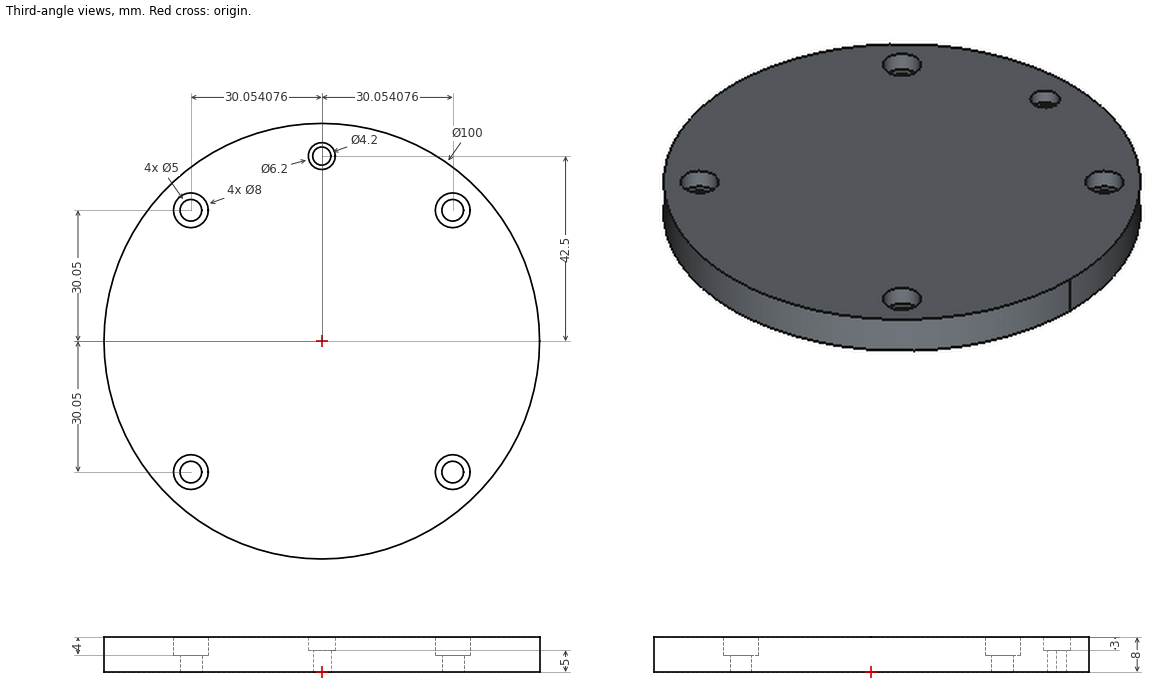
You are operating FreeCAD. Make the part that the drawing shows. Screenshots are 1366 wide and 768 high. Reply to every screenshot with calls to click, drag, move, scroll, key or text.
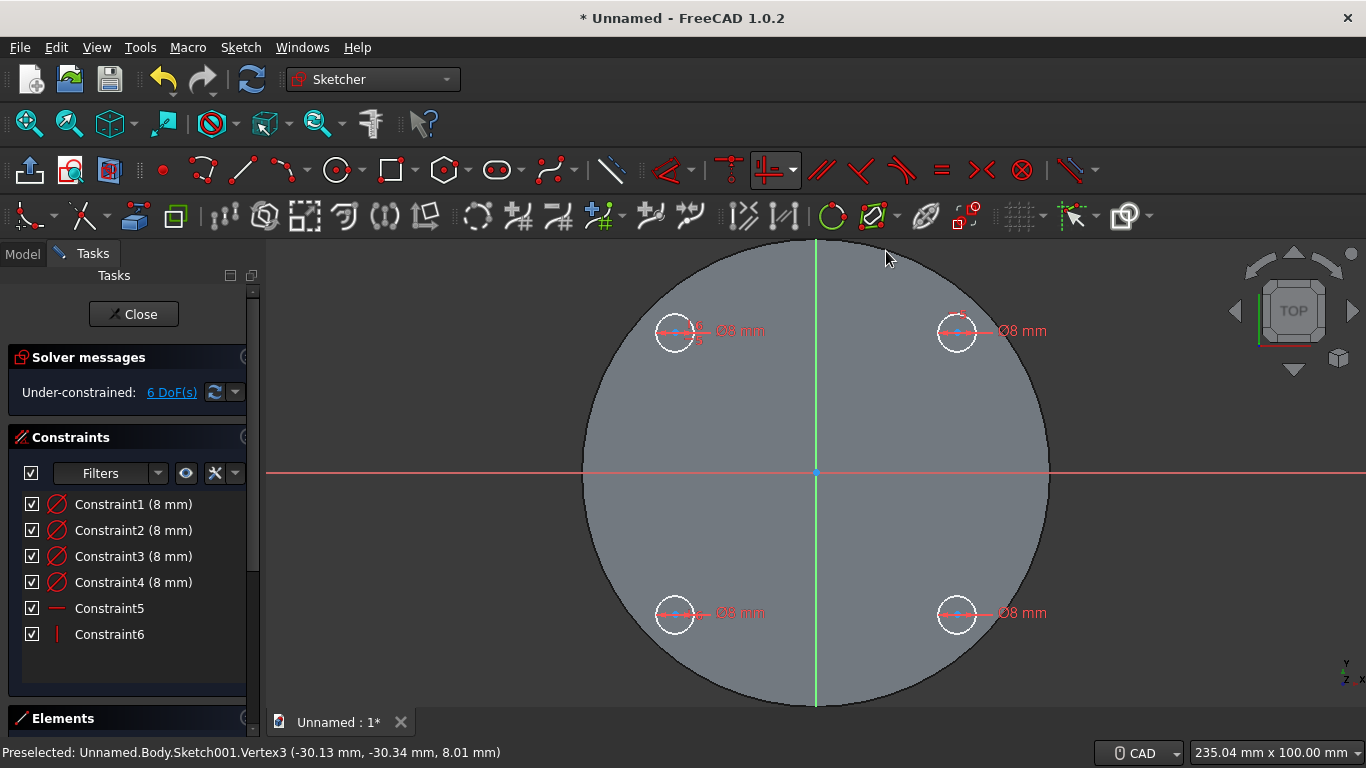
click(957, 333)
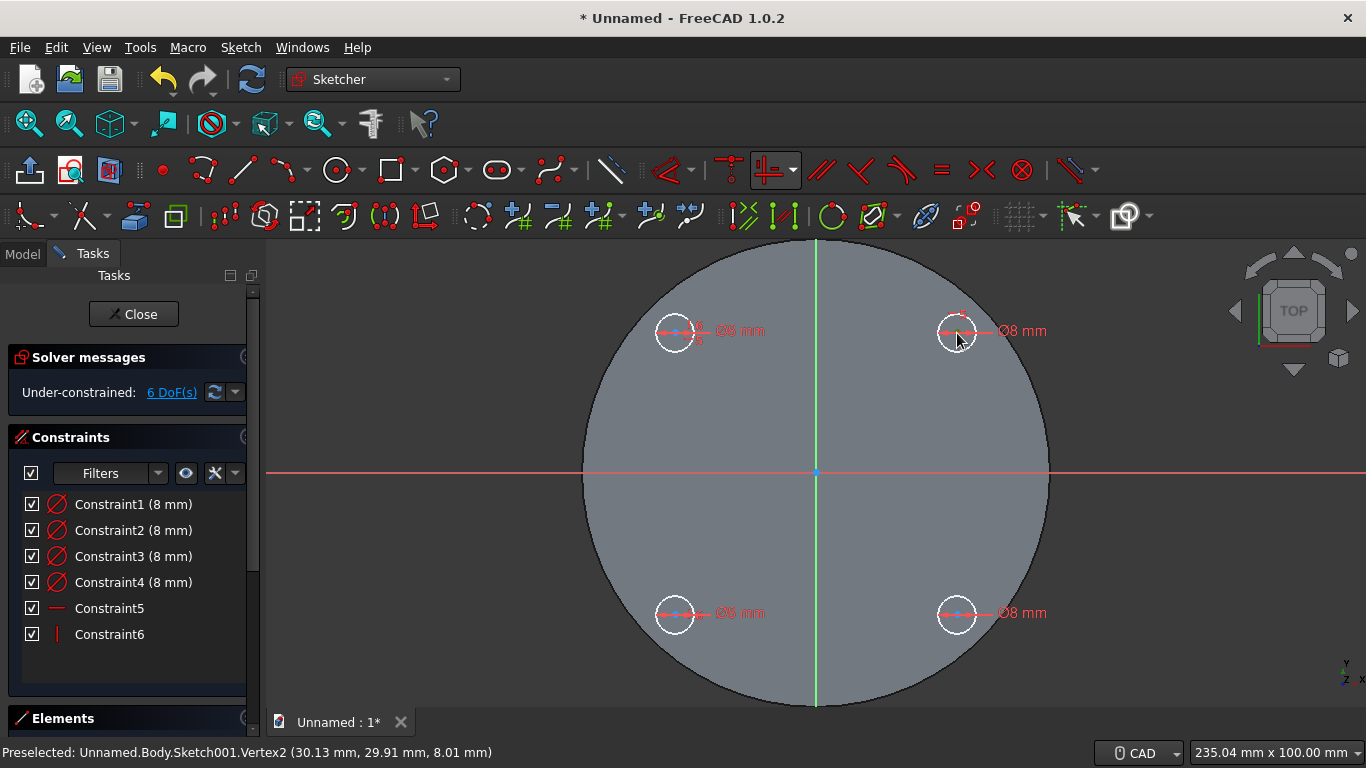
click(957, 615)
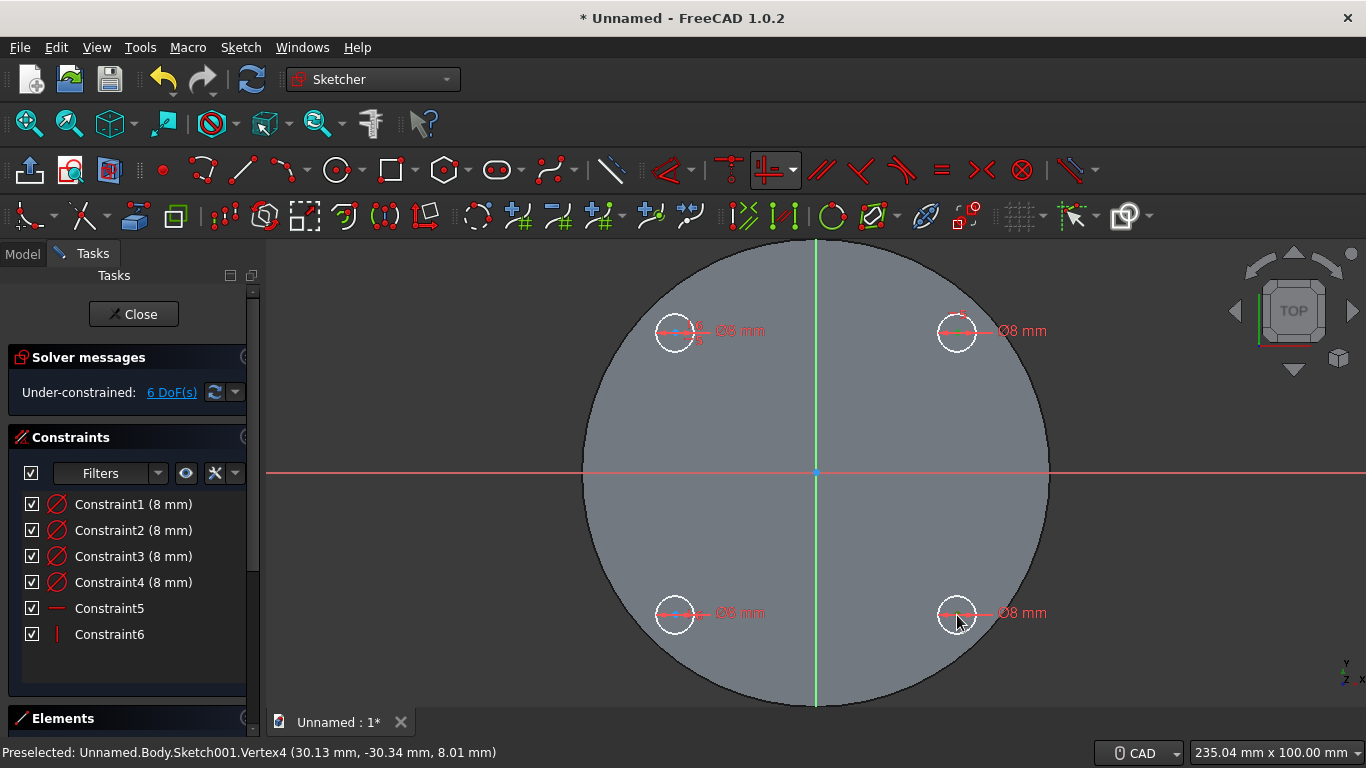
key(v)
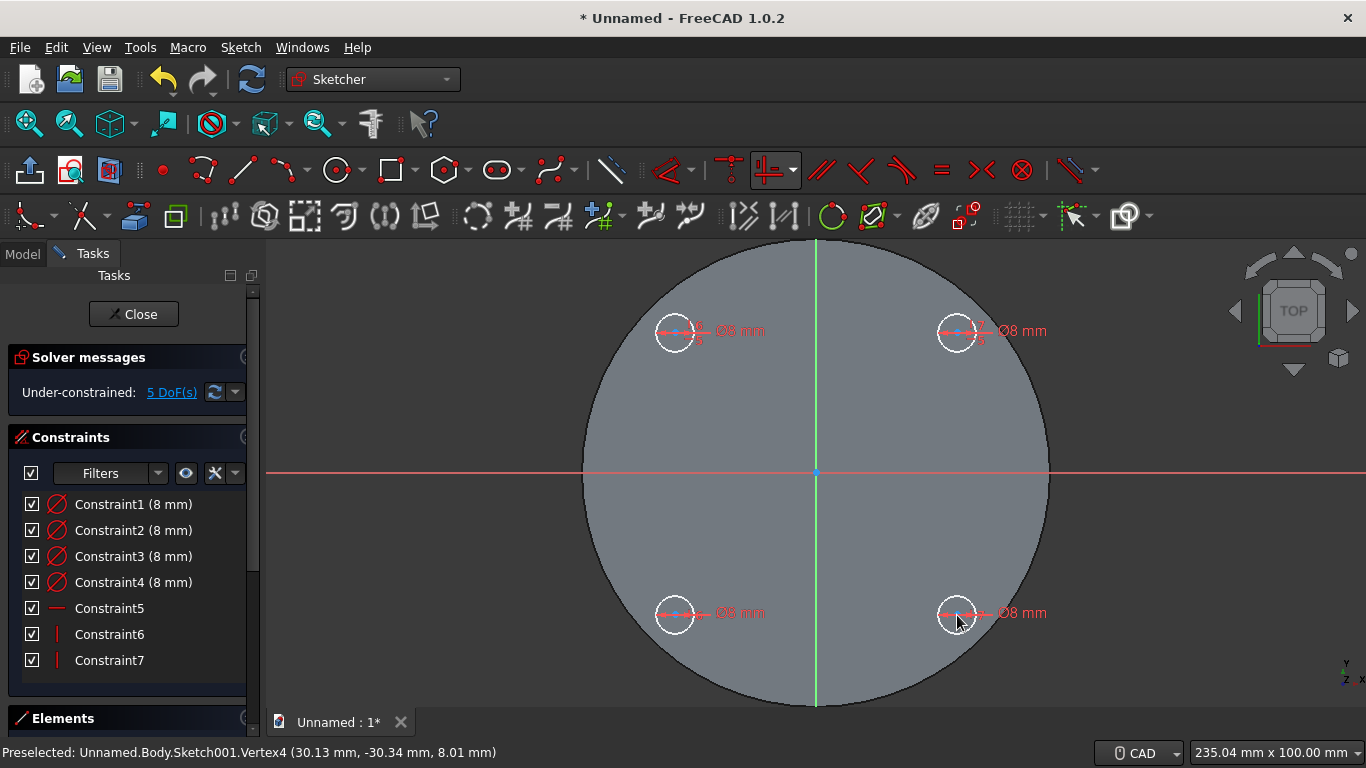
click(675, 615)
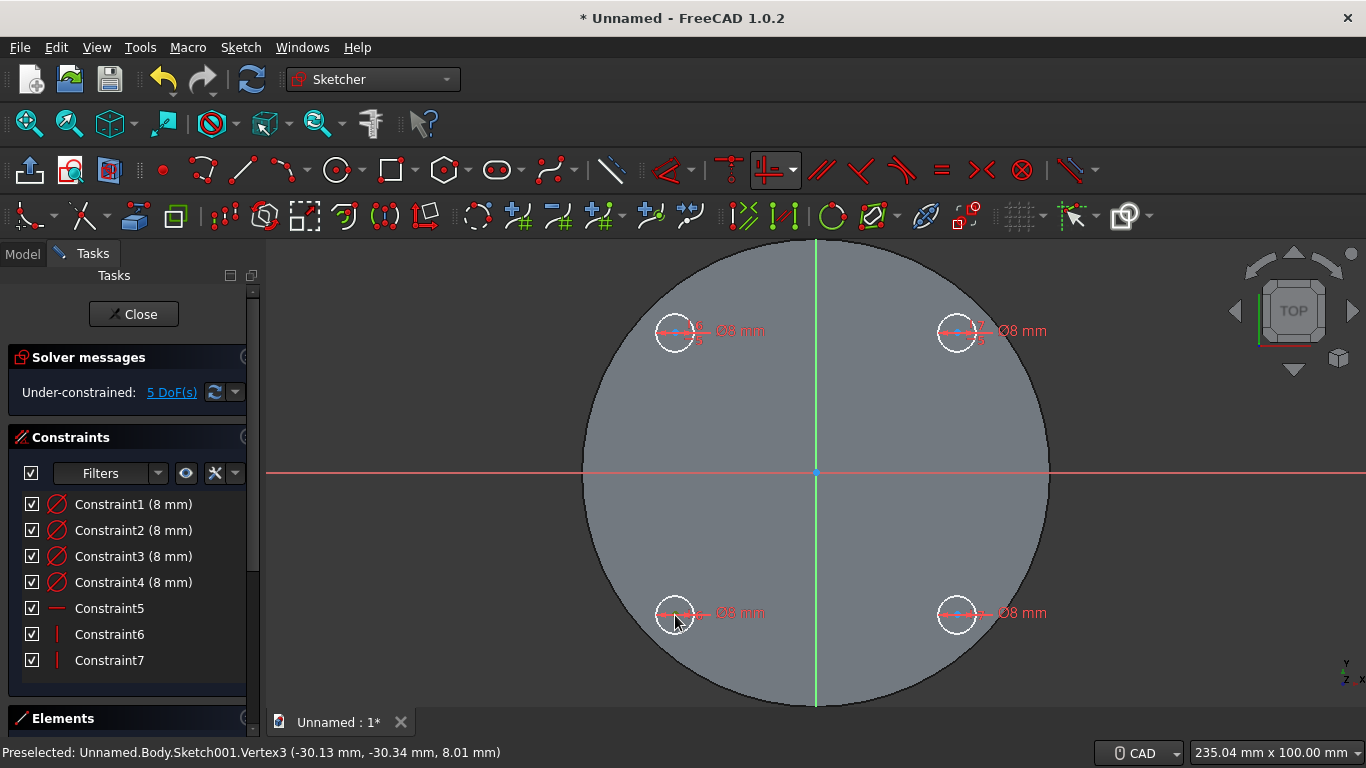
click(957, 615)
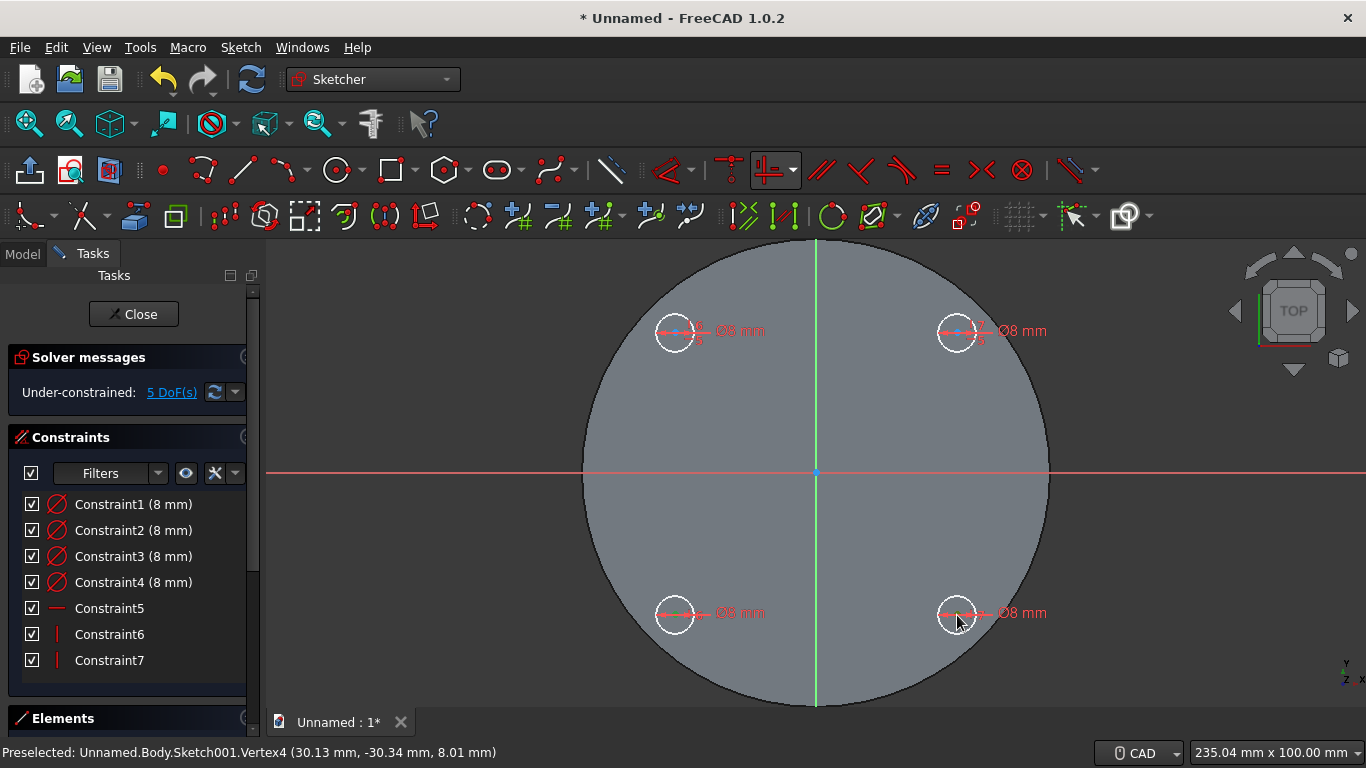
key(h)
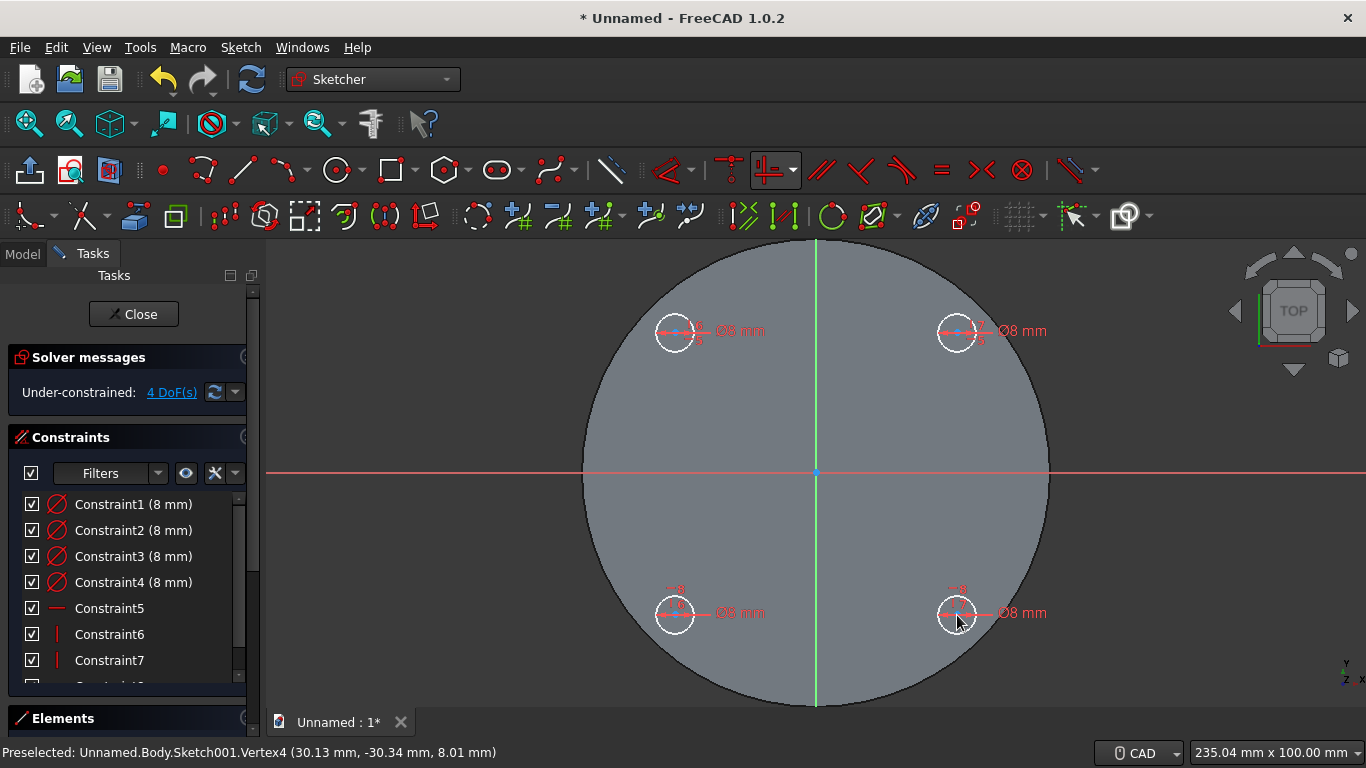
click(675, 333)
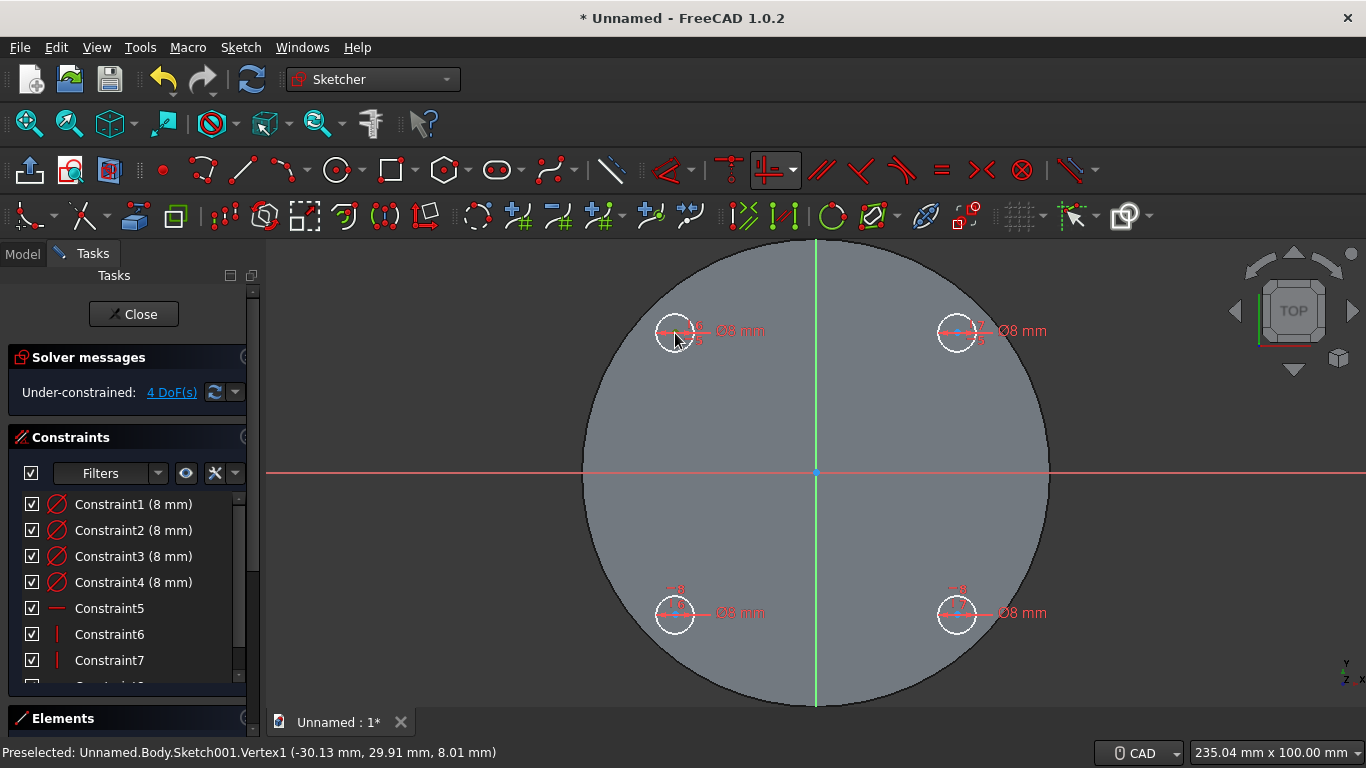
key(i)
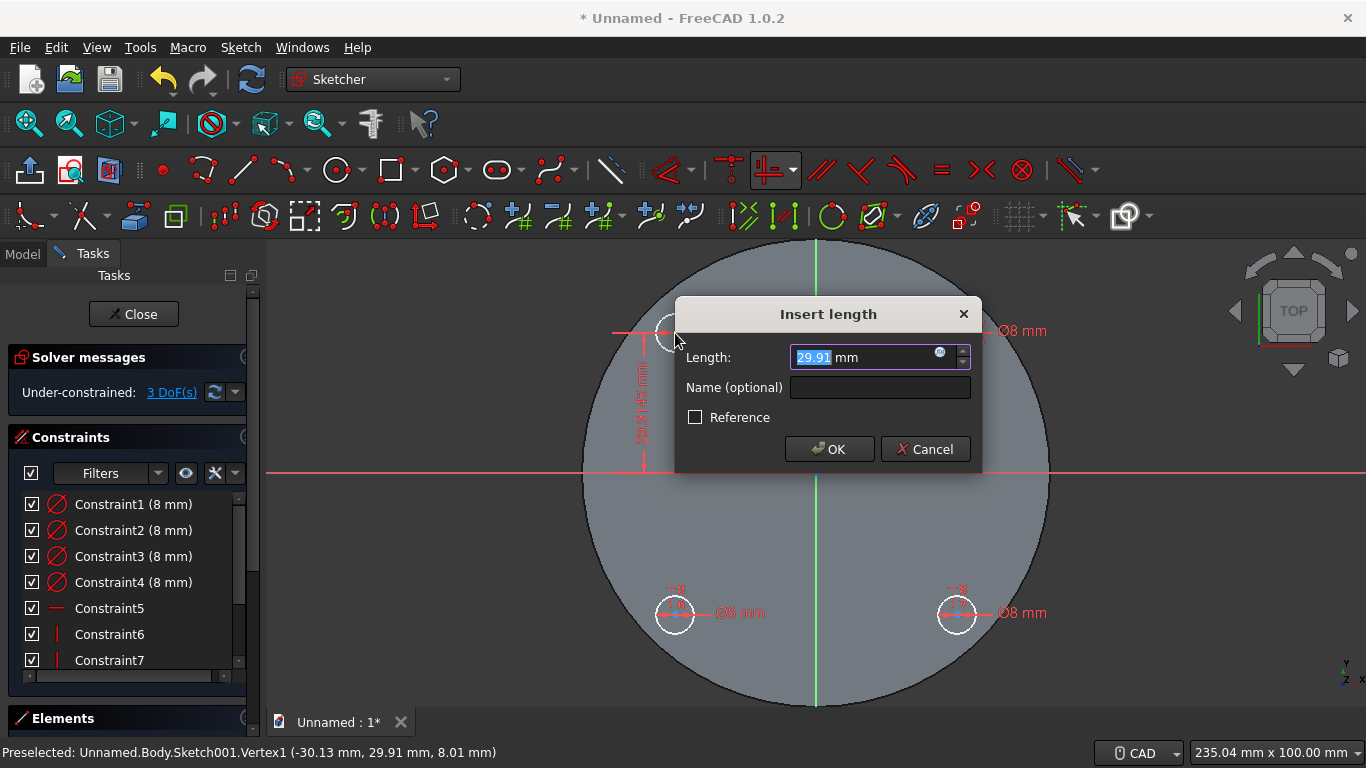
text(30.05)
key(Return)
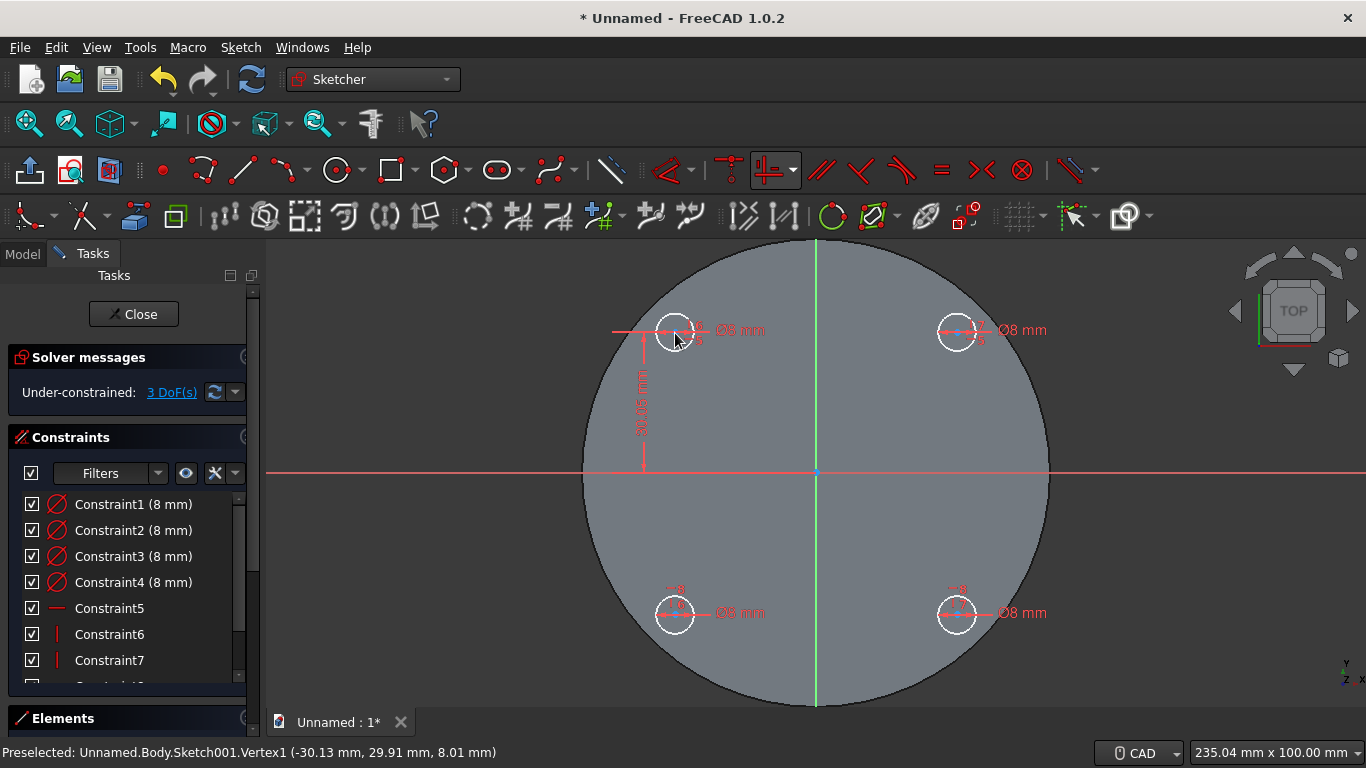
click(675, 615)